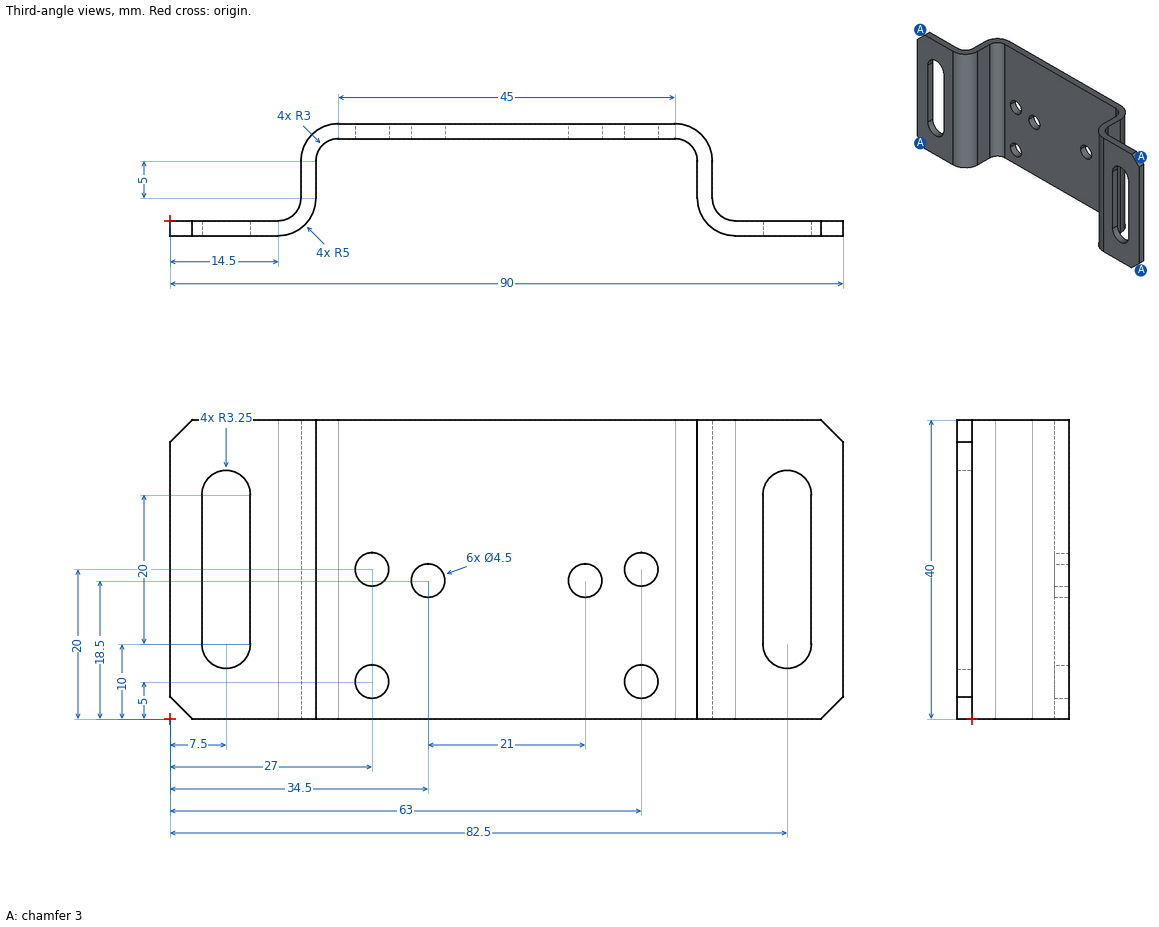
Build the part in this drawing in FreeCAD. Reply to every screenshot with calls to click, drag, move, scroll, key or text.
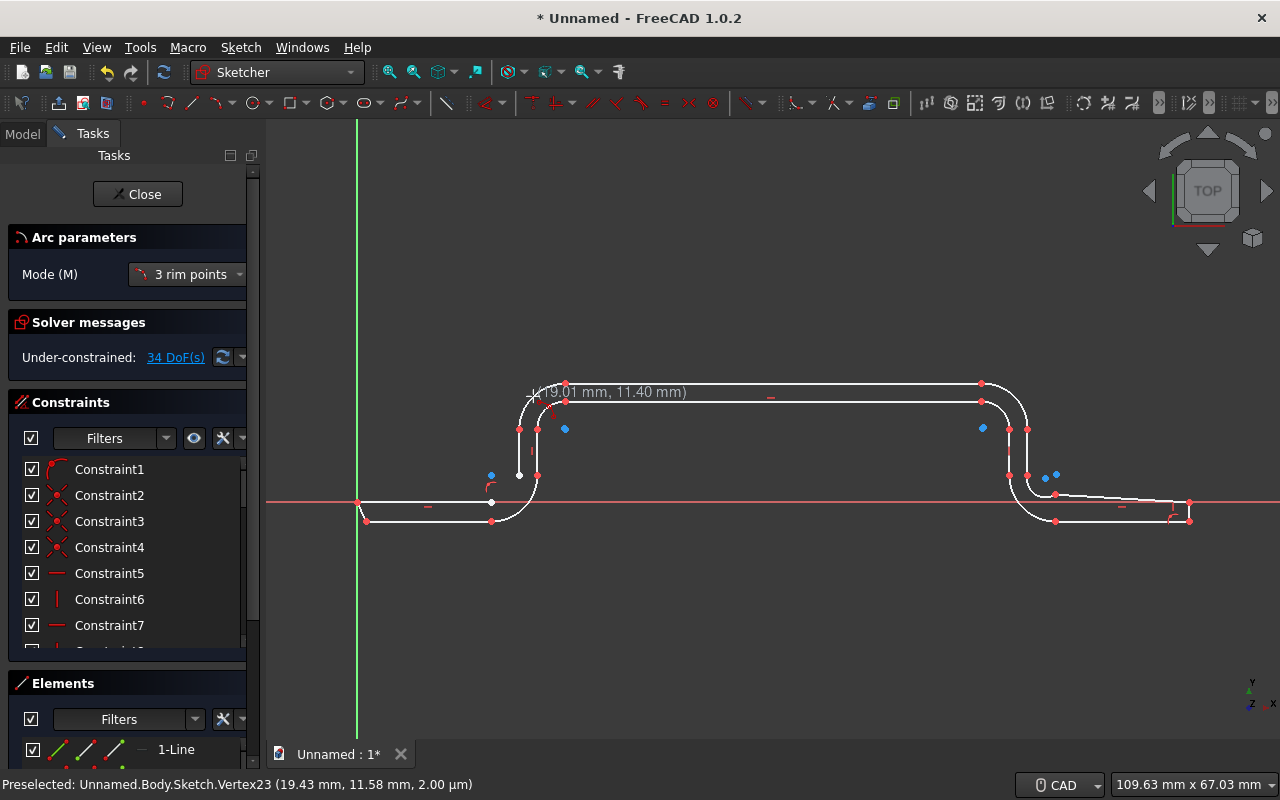
click(519, 476)
click(492, 502)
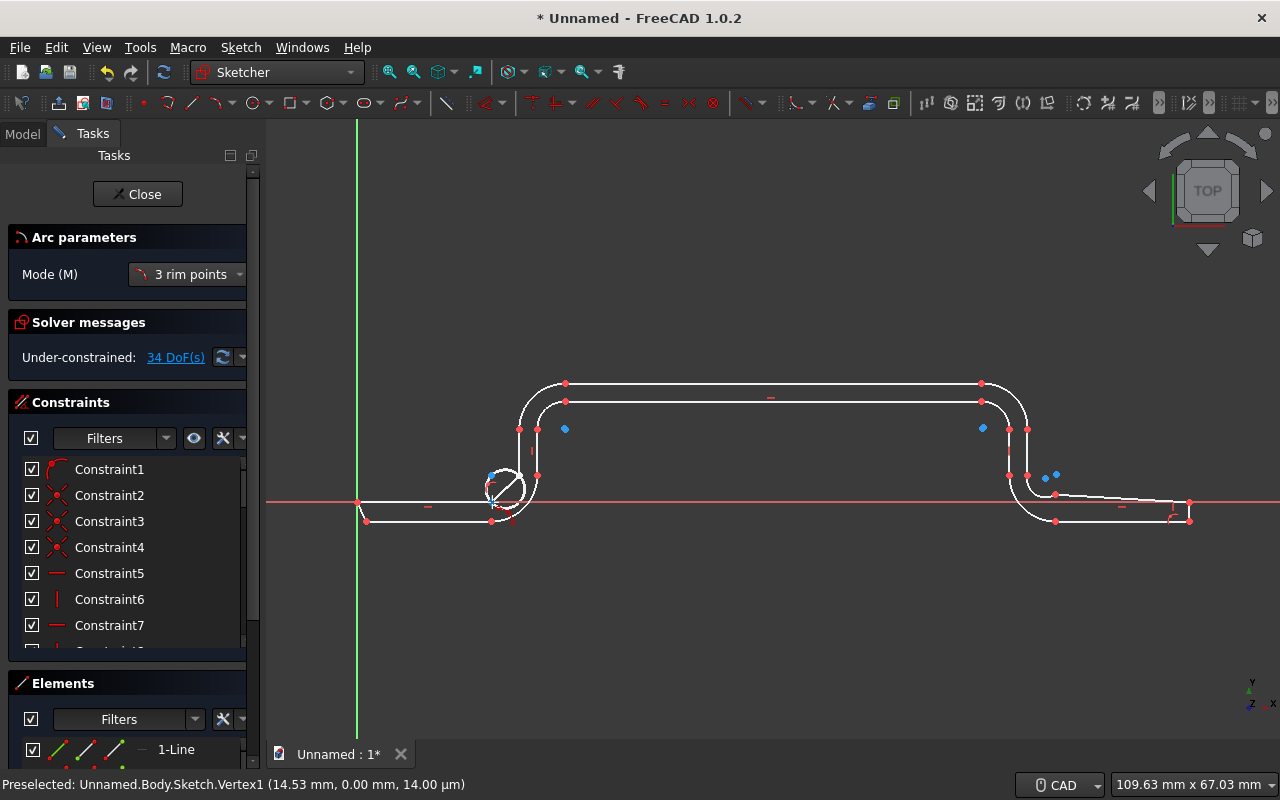
scroll(511, 494, up, 4)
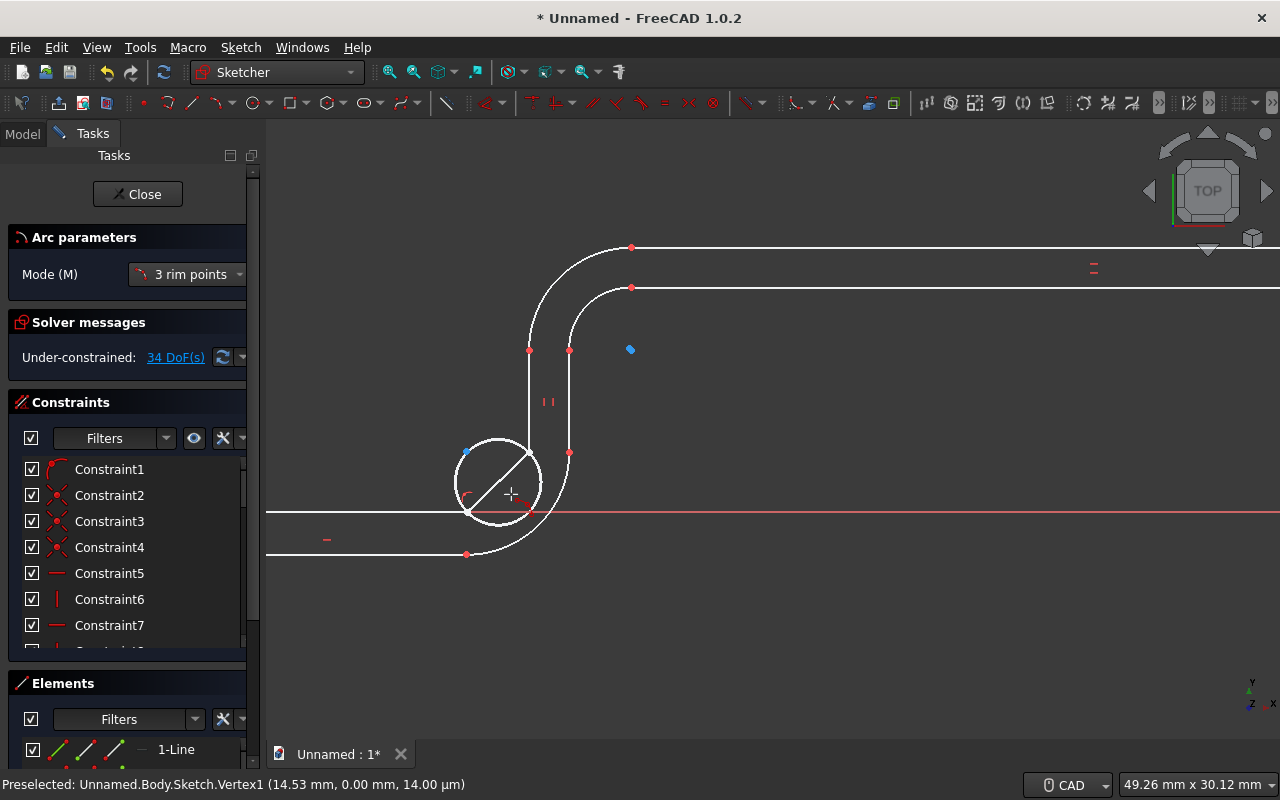
click(510, 494)
key(Escape)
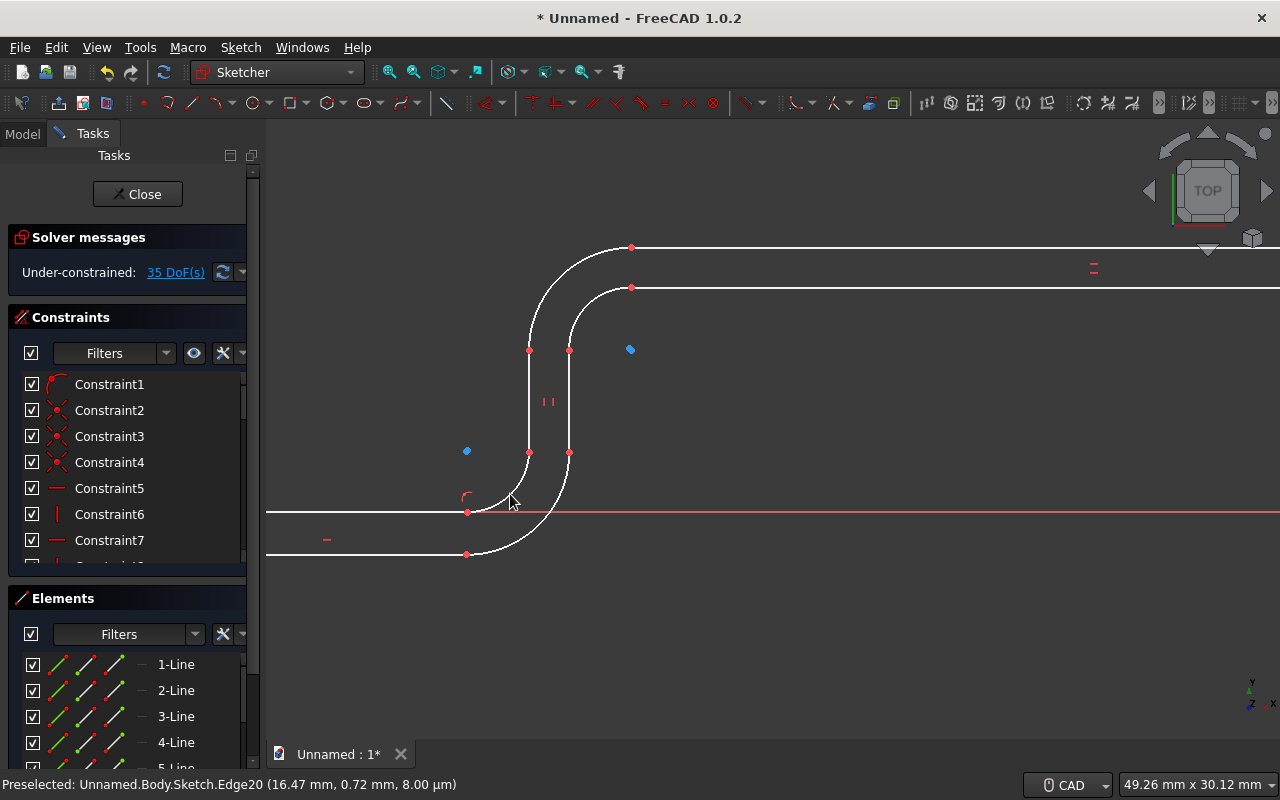
click(378, 512)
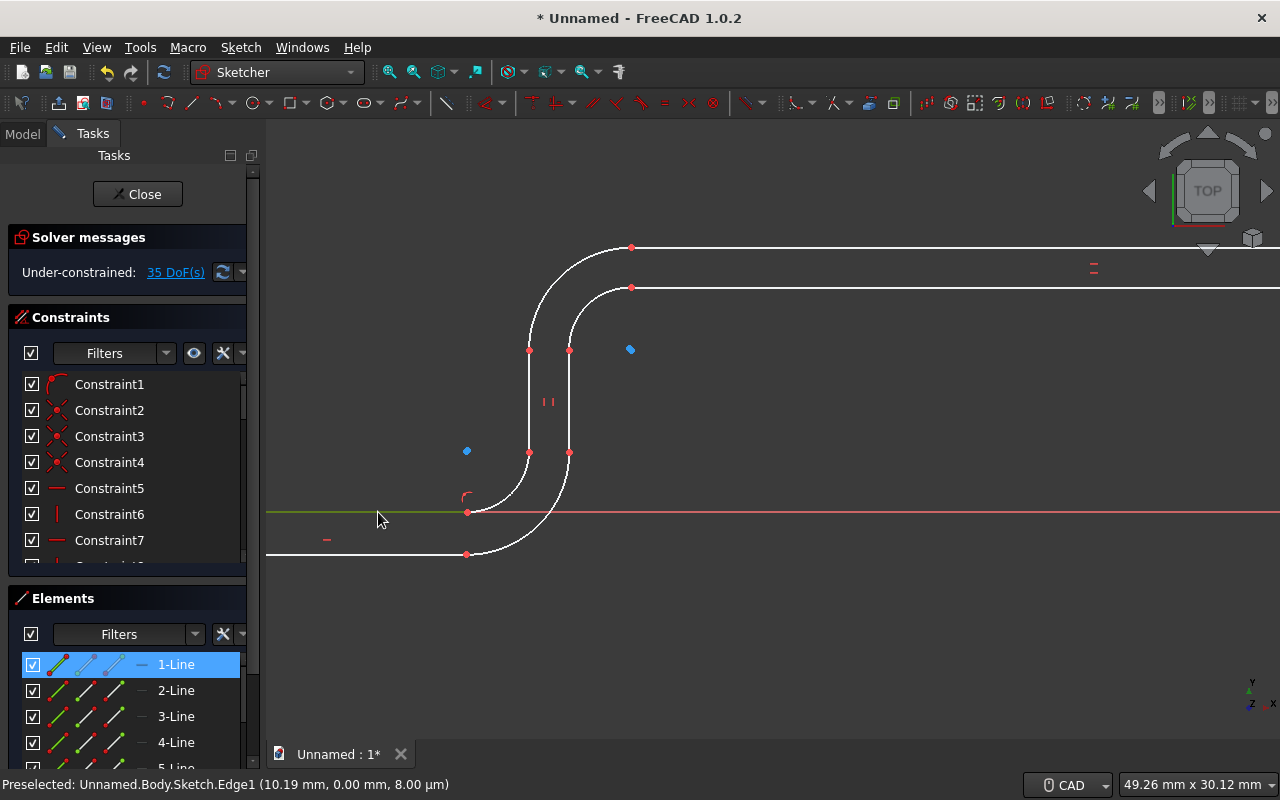
click(522, 480)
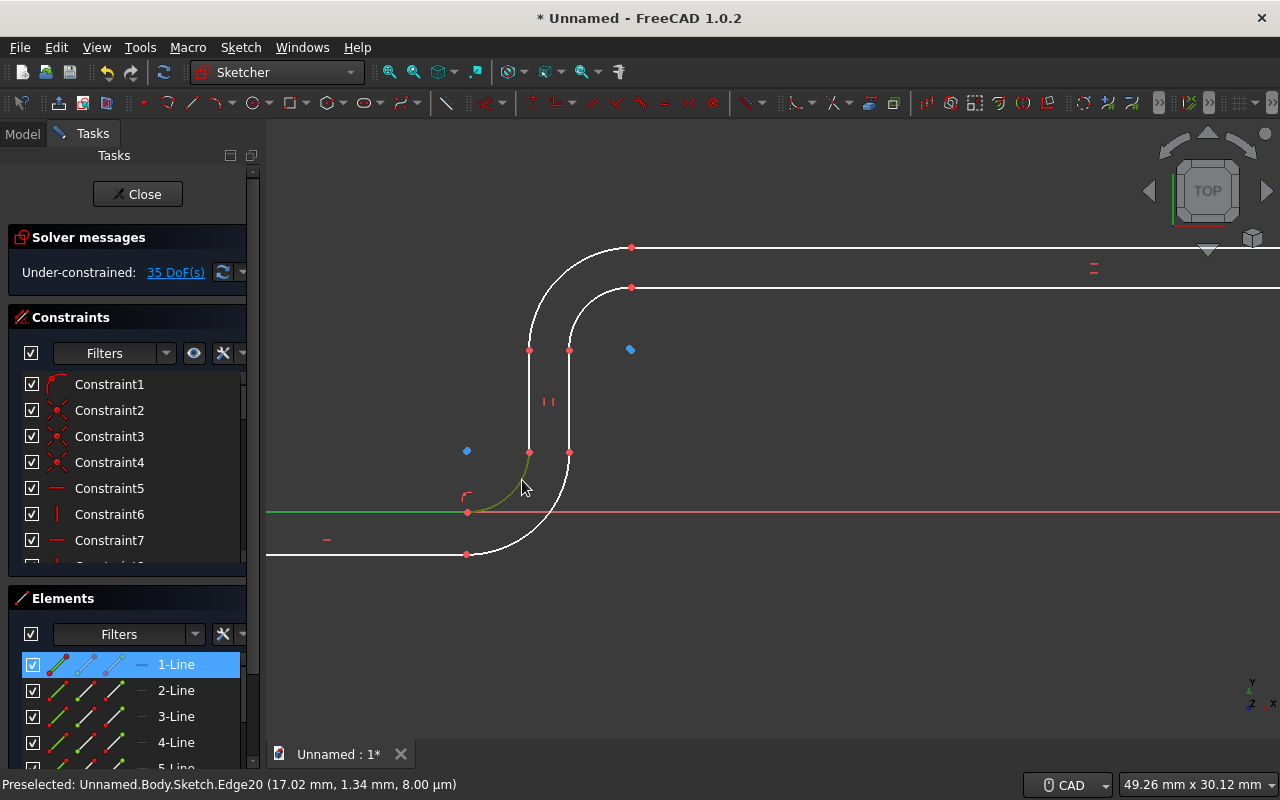
key(t)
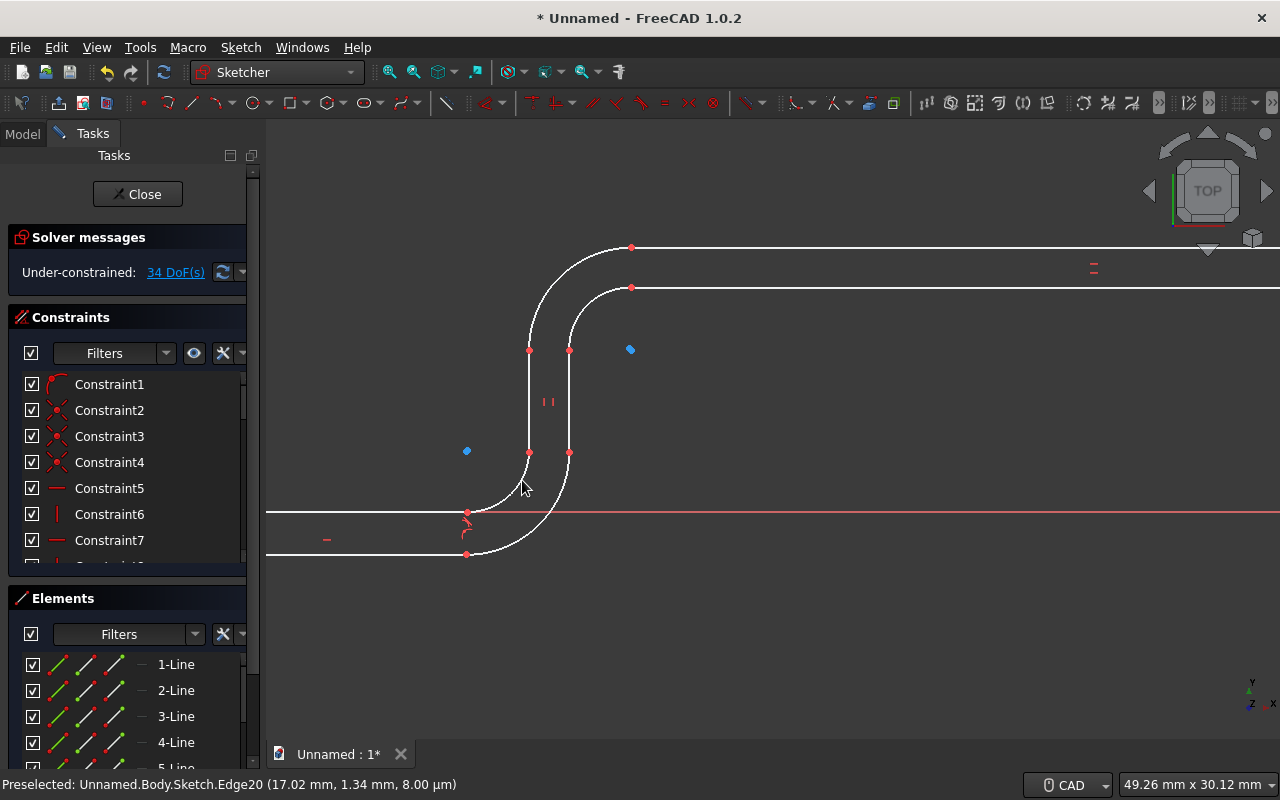
click(383, 555)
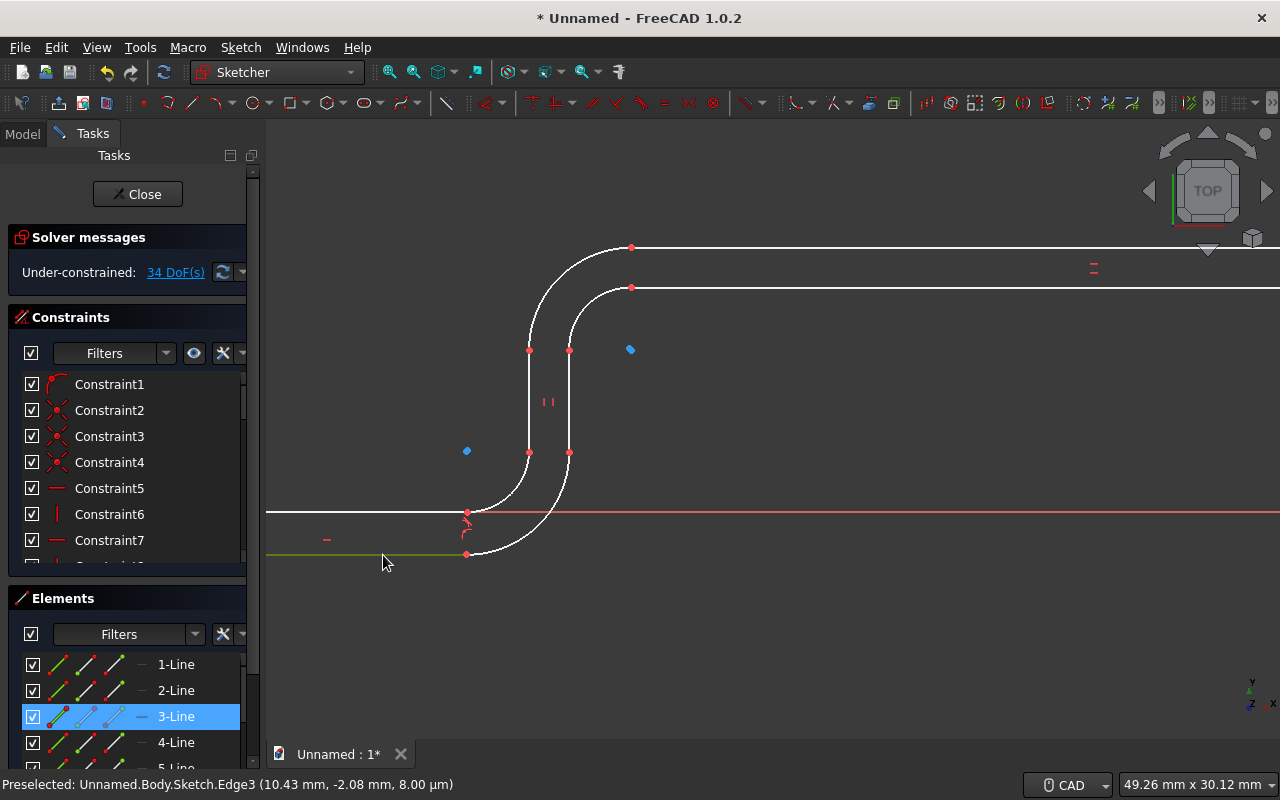
click(513, 544)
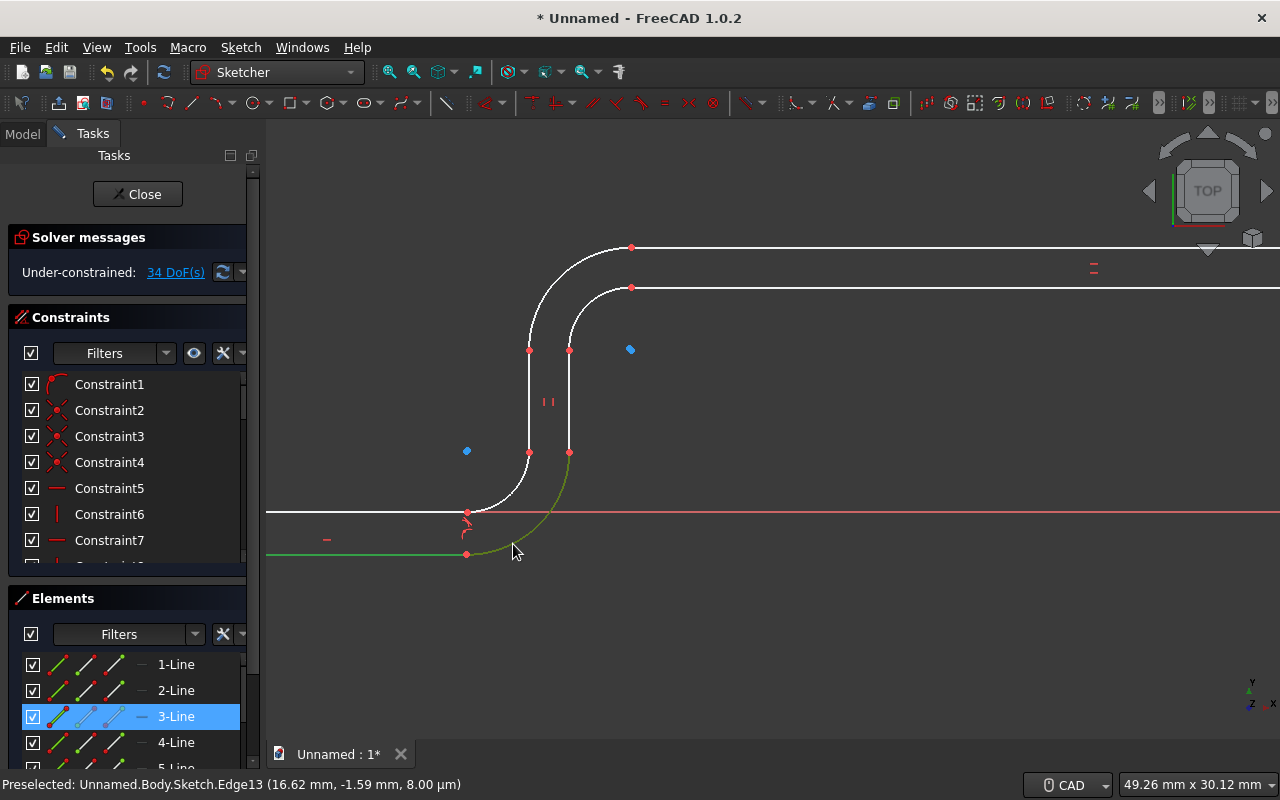
key(t)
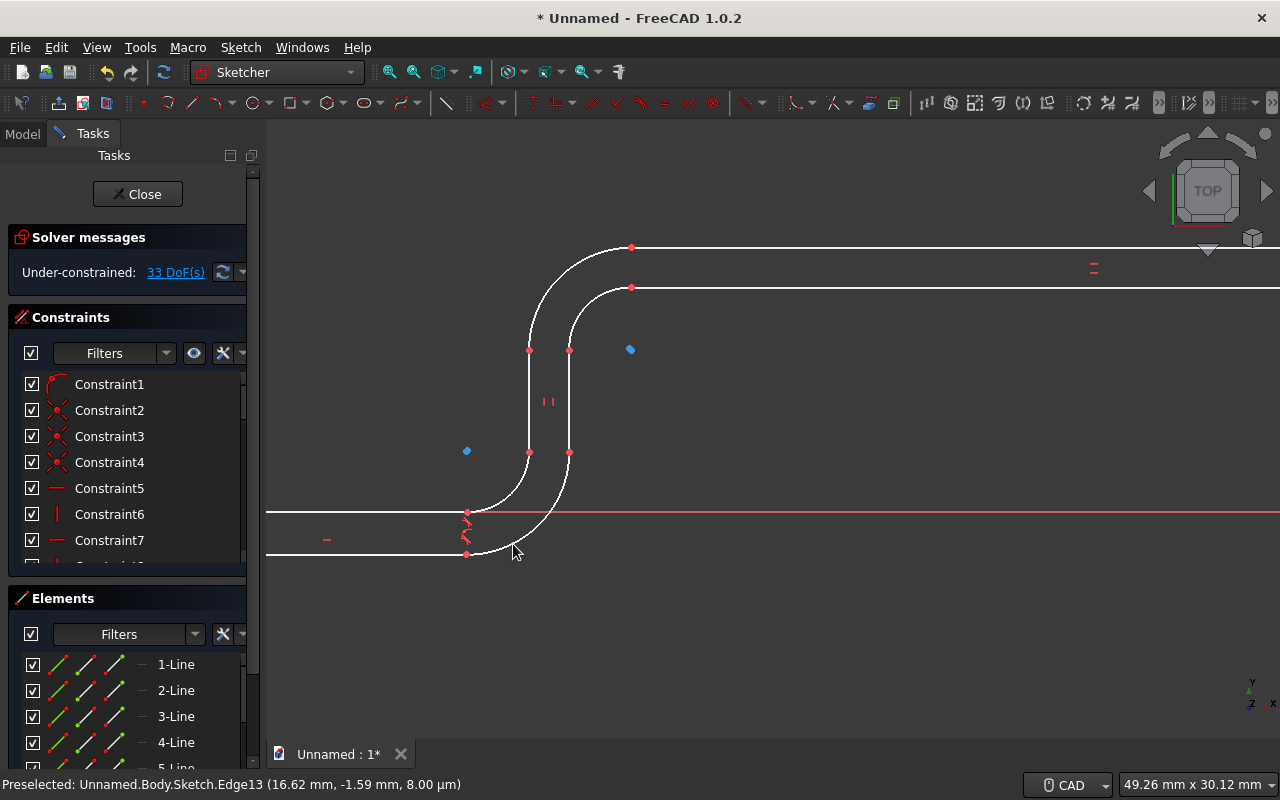
click(569, 422)